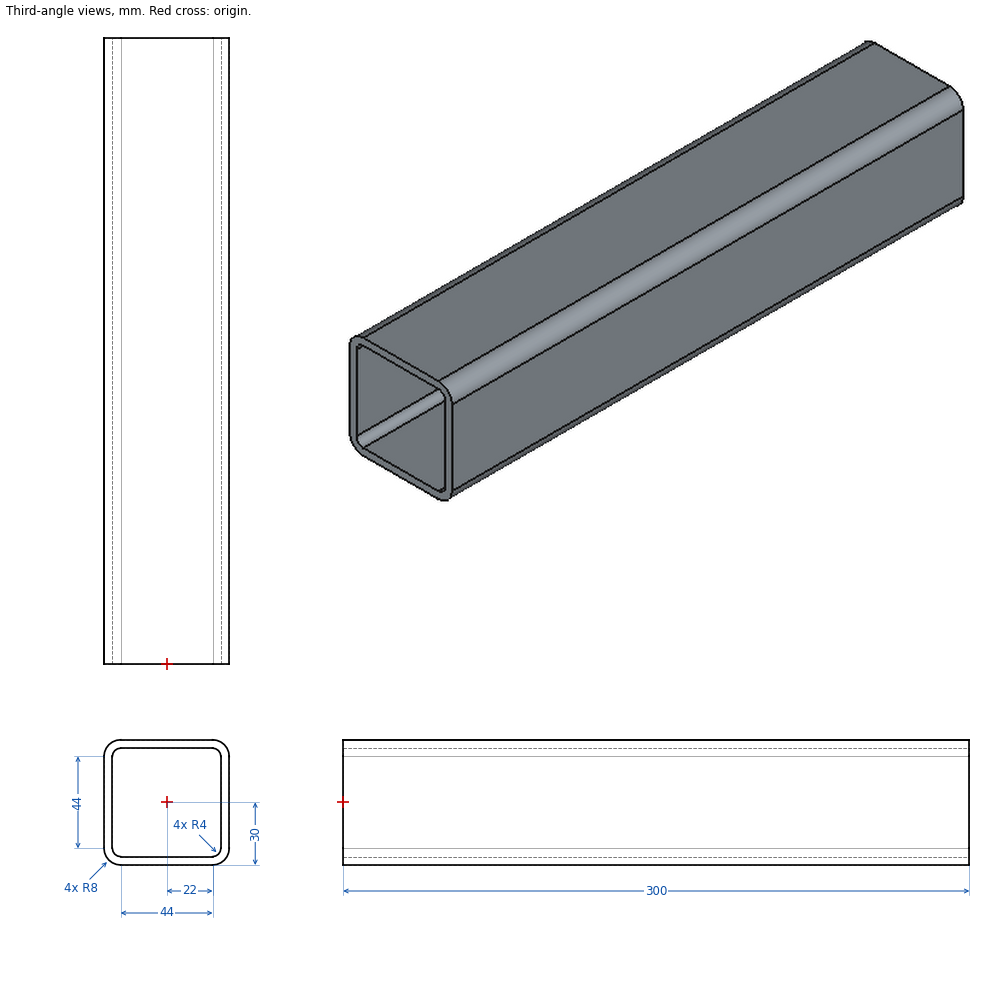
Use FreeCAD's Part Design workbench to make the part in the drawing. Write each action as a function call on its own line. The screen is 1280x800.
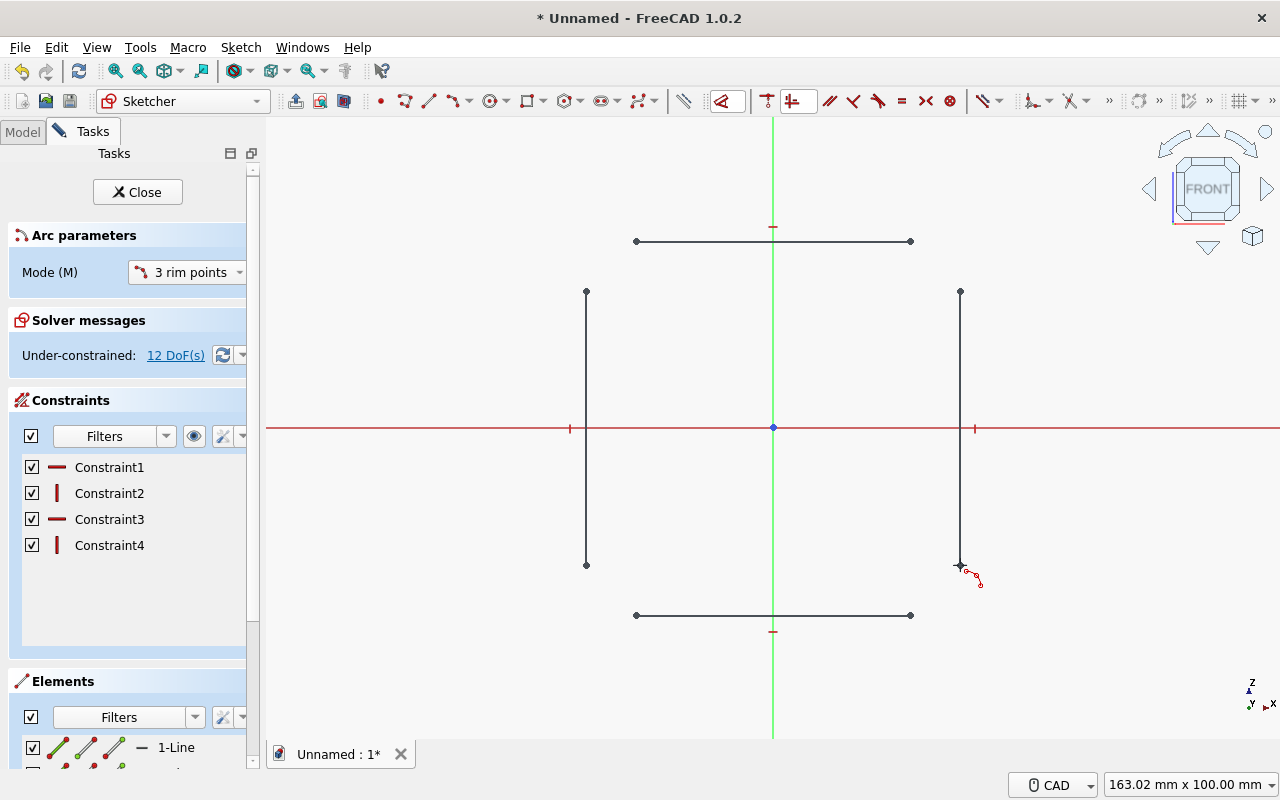
click(636, 616)
click(586, 566)
click(601, 600)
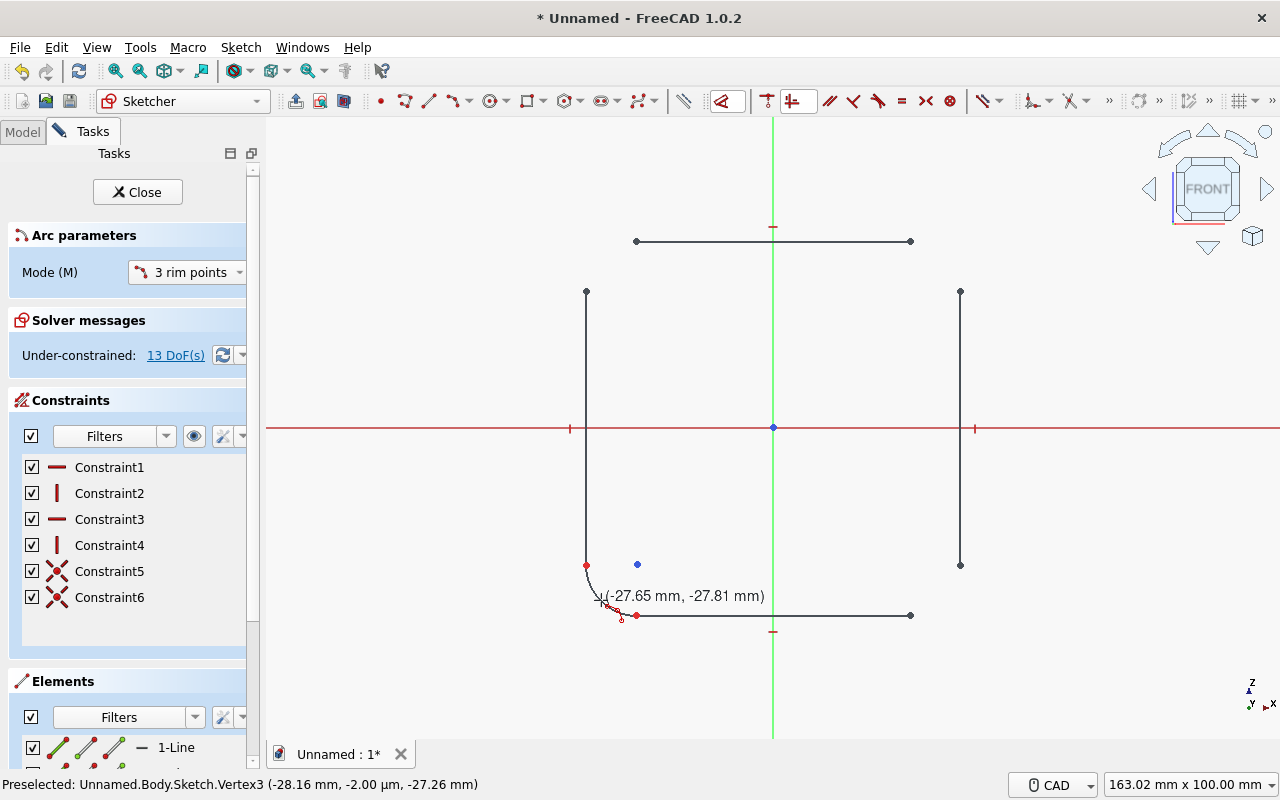
click(586, 292)
click(636, 242)
click(601, 256)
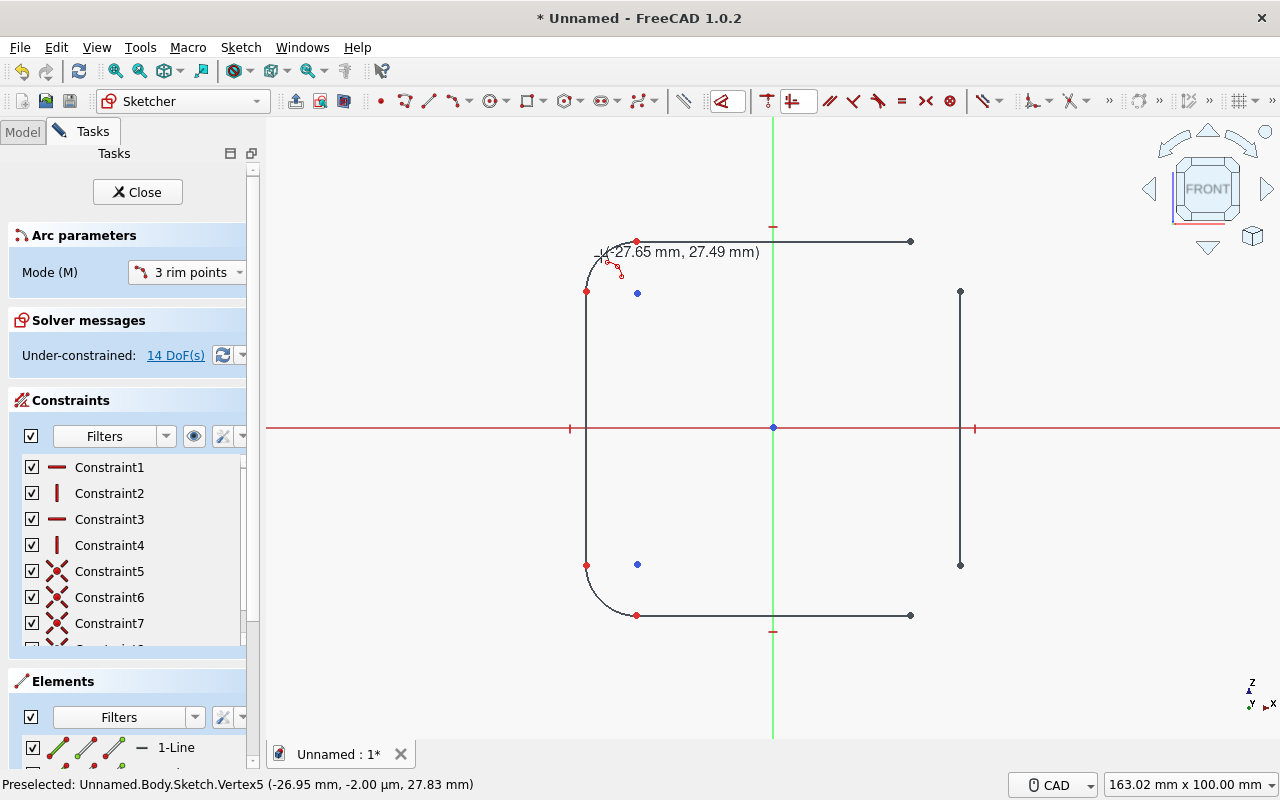
click(910, 242)
click(960, 292)
click(945, 256)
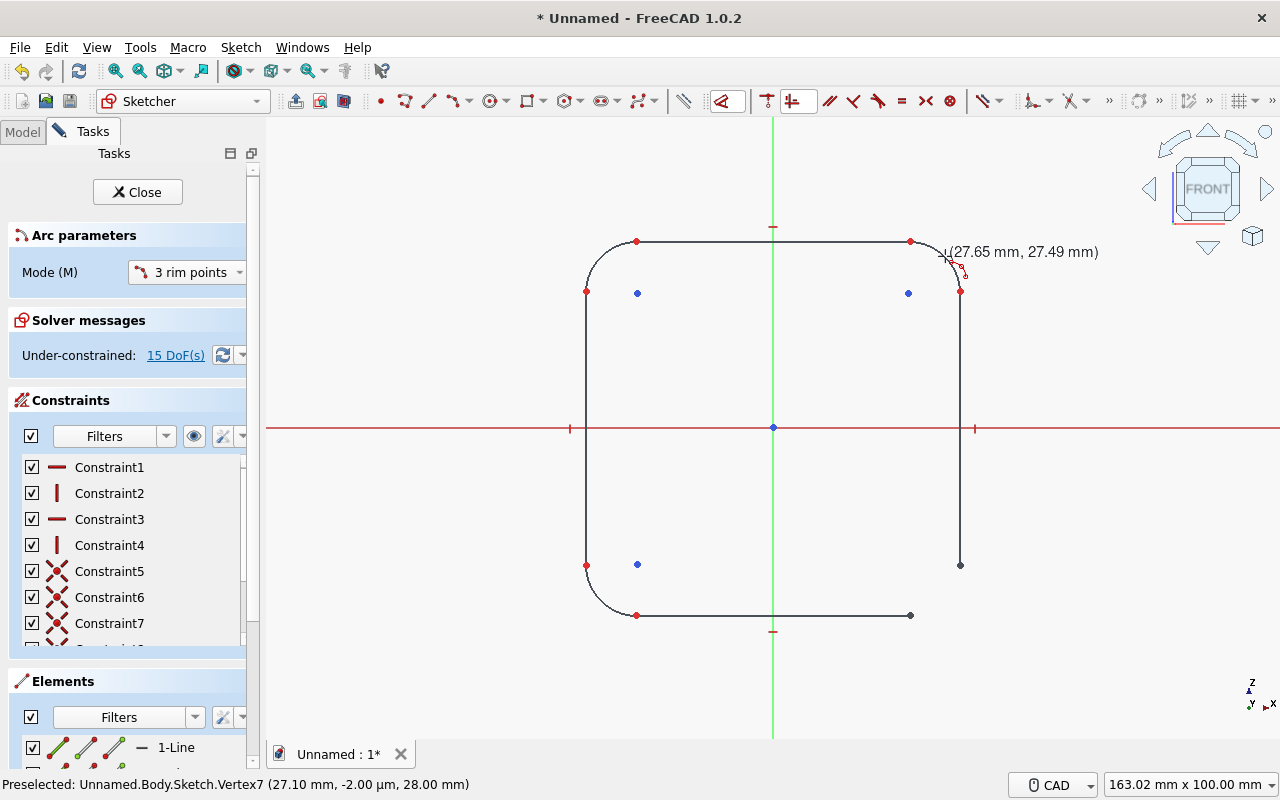
click(960, 566)
click(910, 616)
click(945, 600)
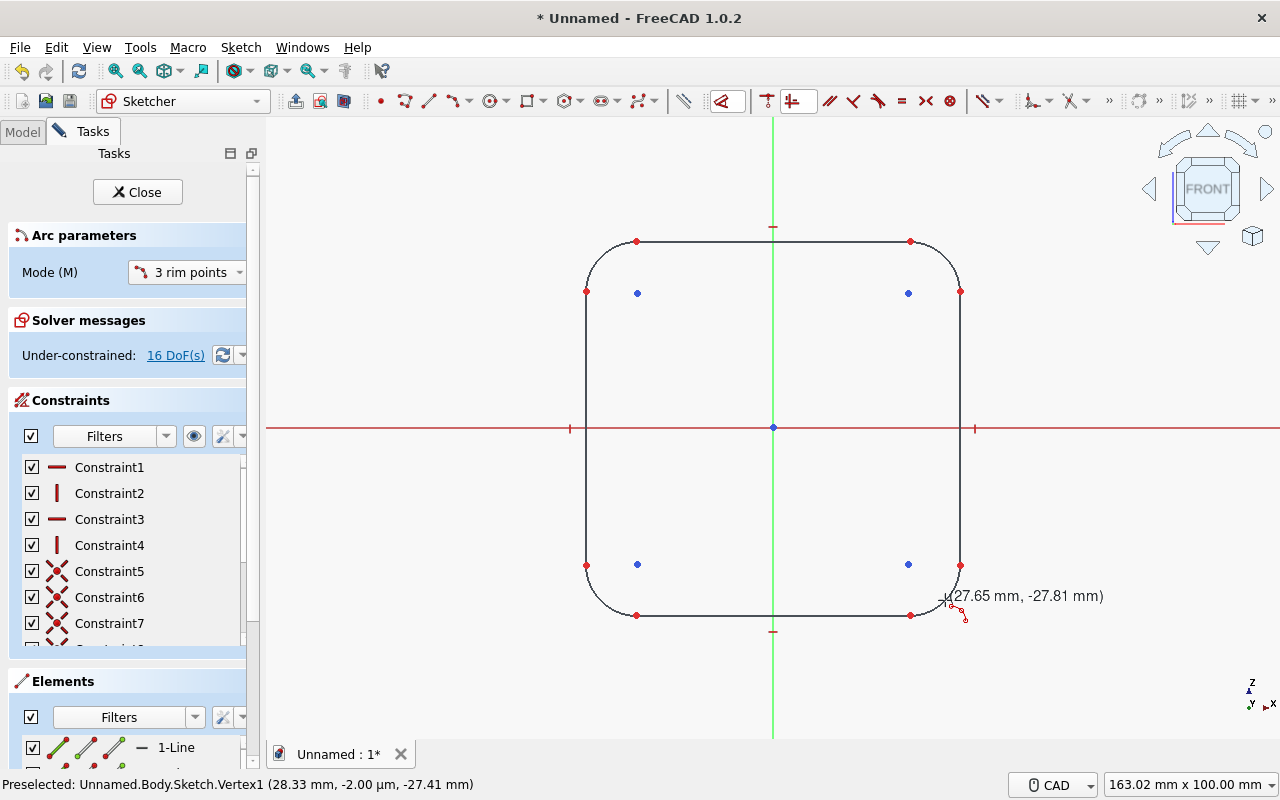
click(430, 102)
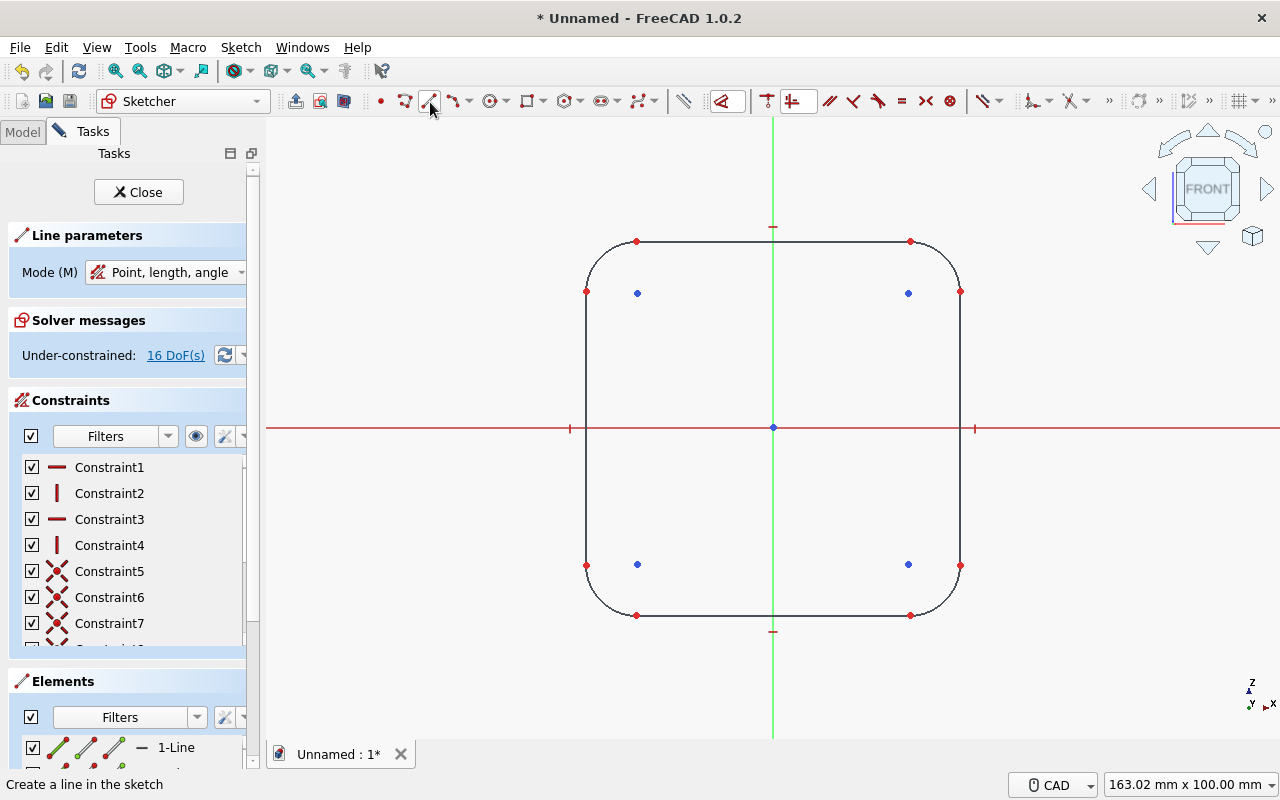
click(636, 590)
click(910, 590)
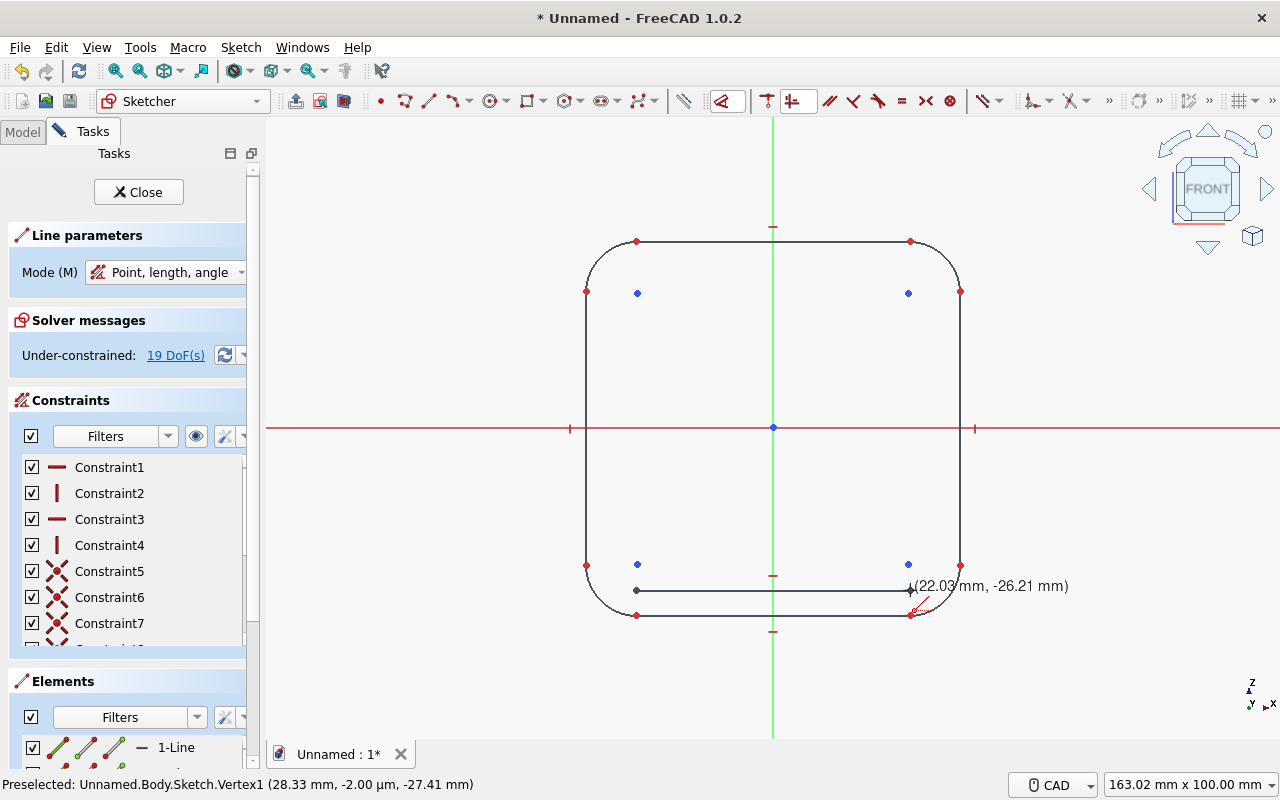
click(935, 565)
click(935, 291)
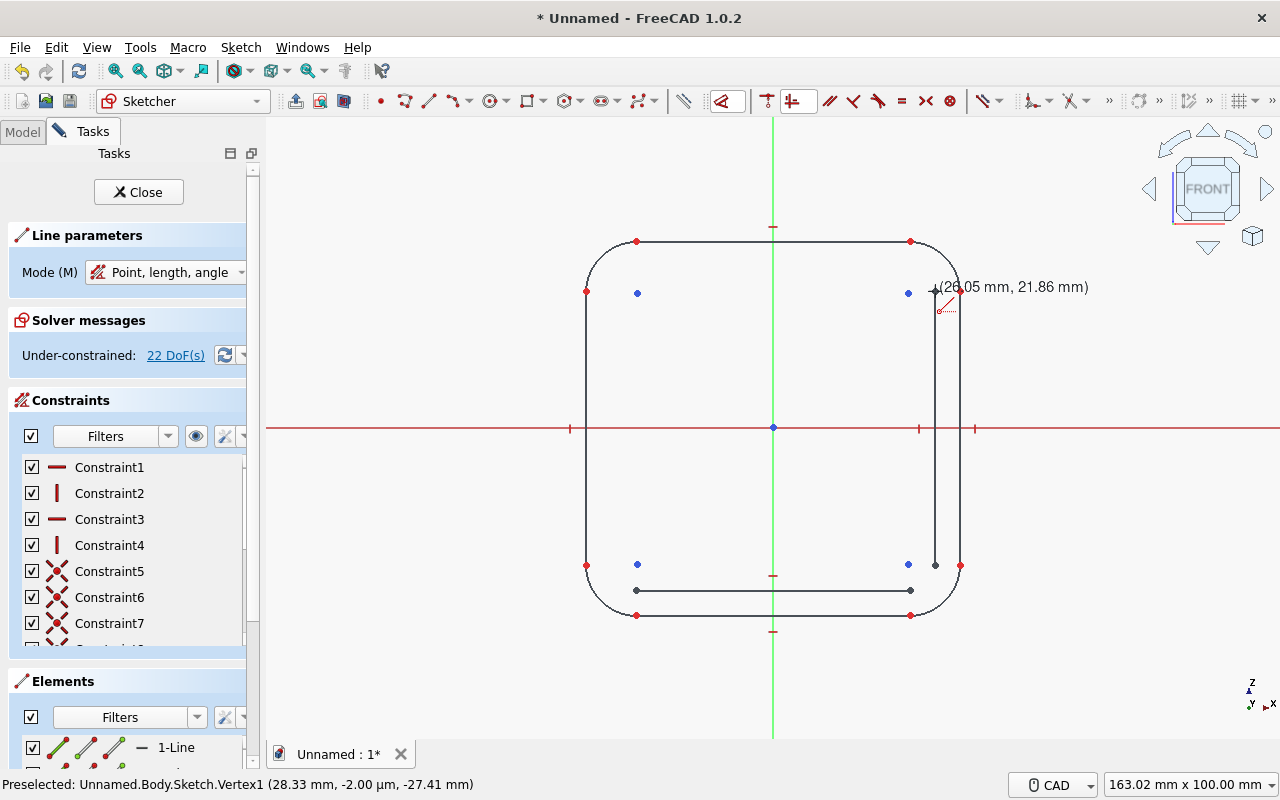
click(910, 266)
click(636, 266)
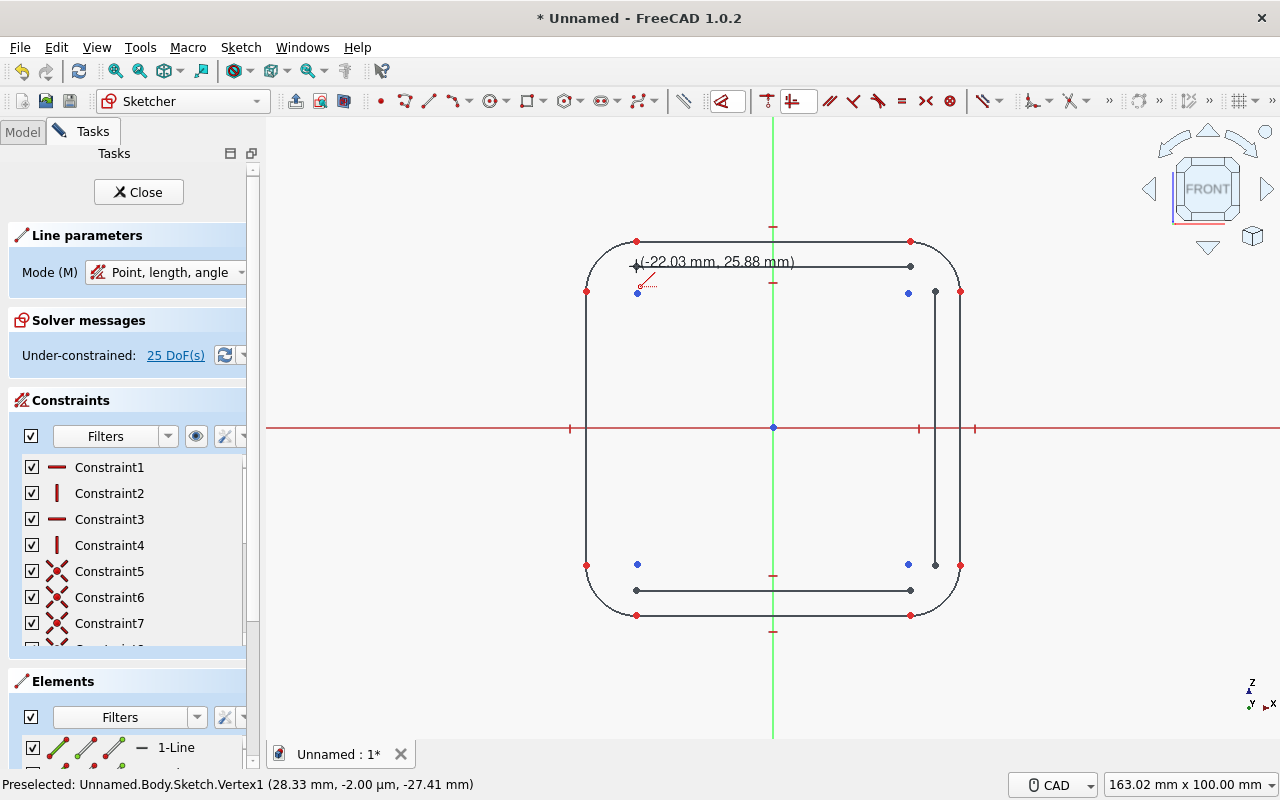
click(611, 291)
click(611, 565)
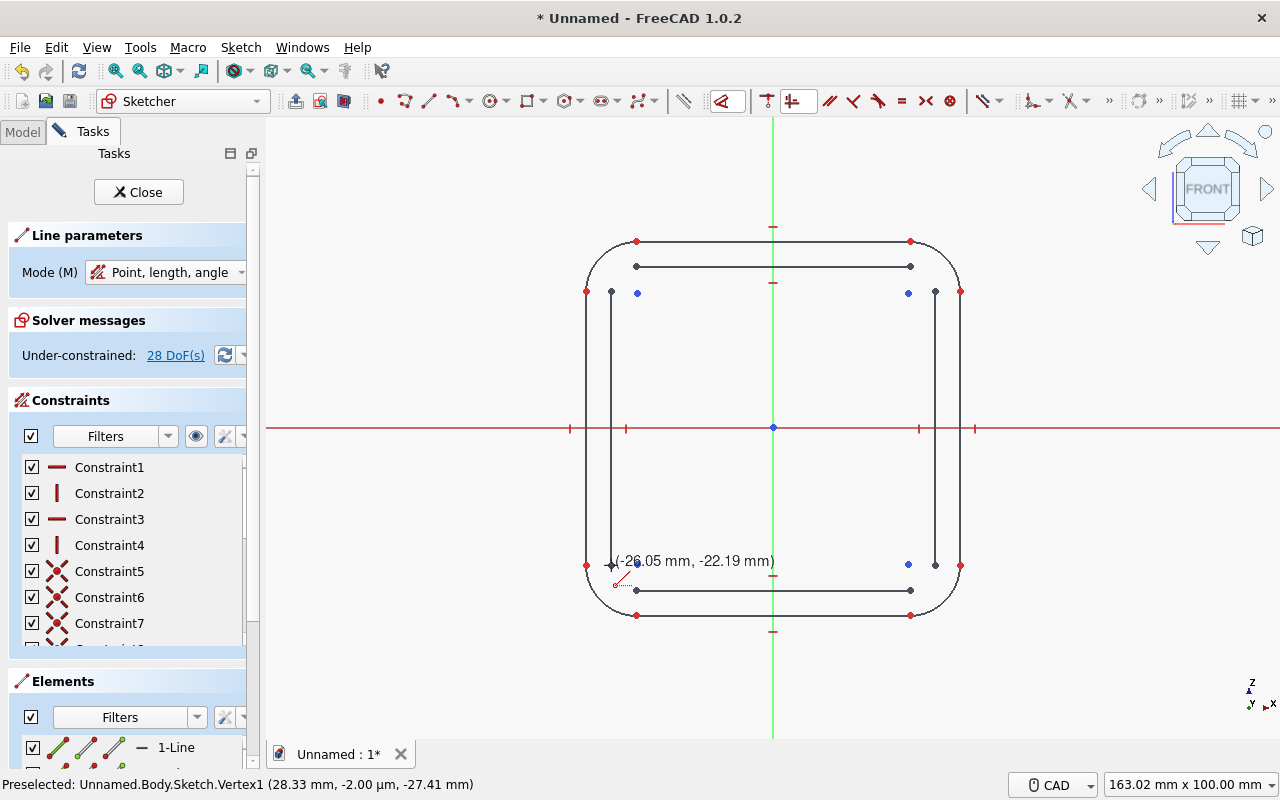
key(g)
key(3)
key(a)